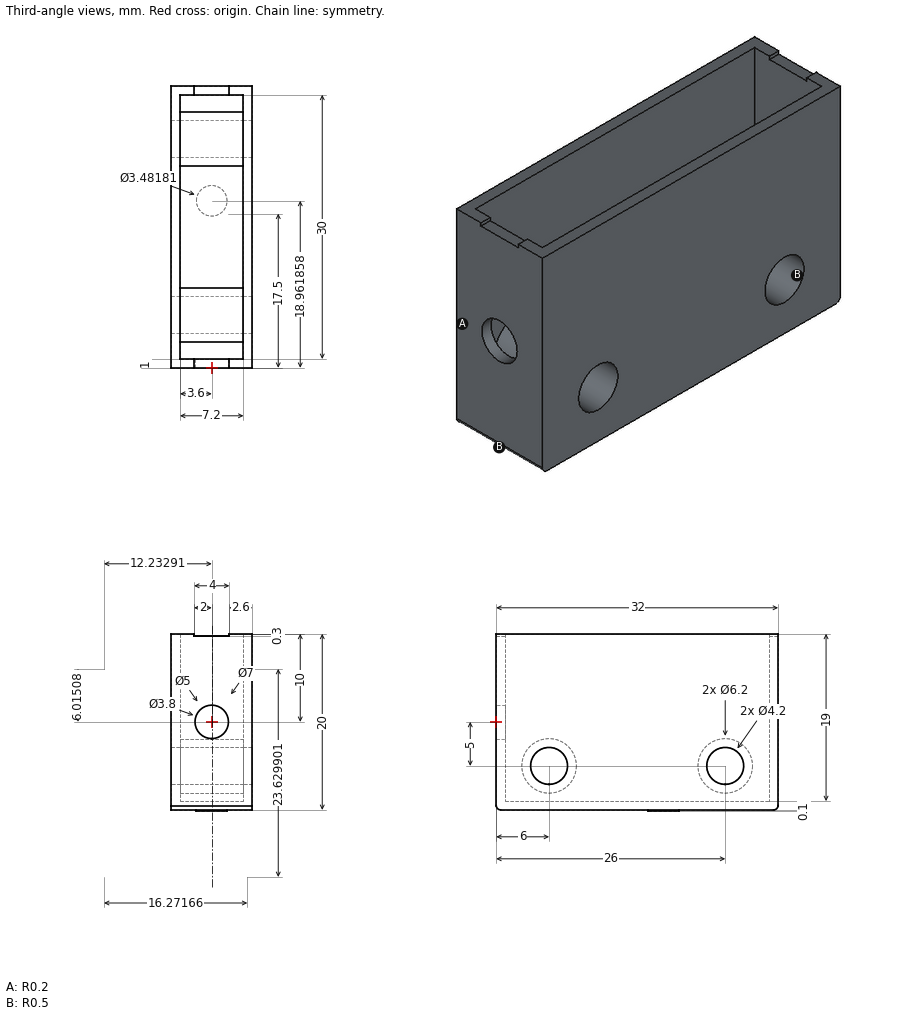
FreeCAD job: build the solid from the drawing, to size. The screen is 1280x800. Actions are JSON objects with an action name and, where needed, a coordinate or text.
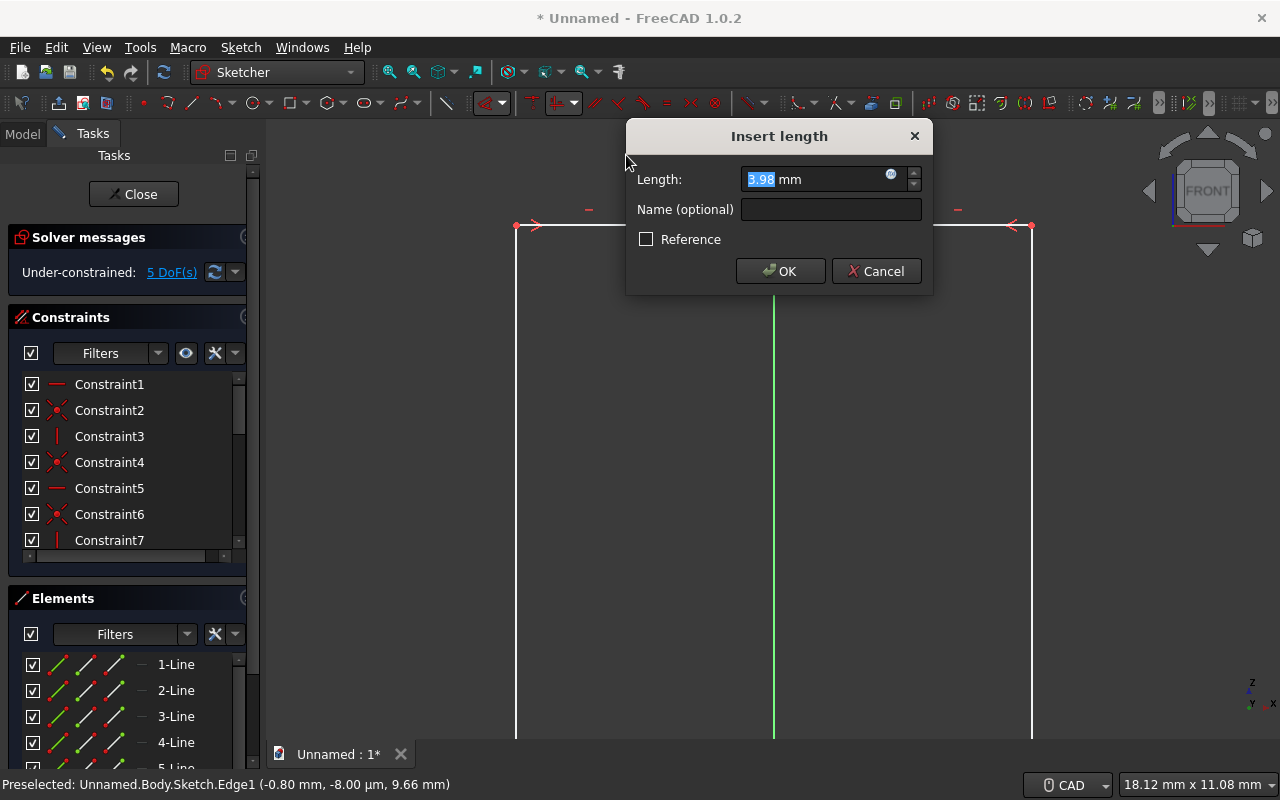
{"action": "type", "text": "4"}
{"action": "key", "text": "Return"}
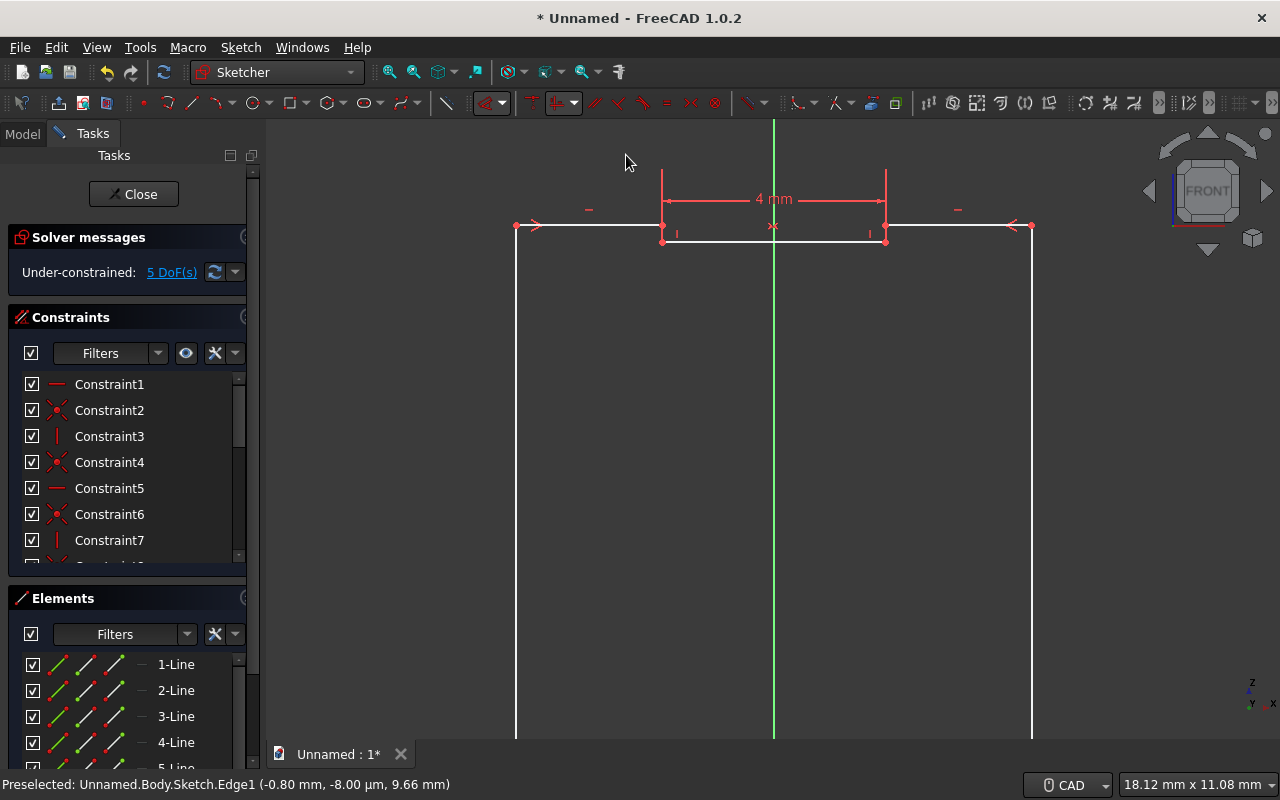
{"action": "left_click", "coordinate": [1032, 561]}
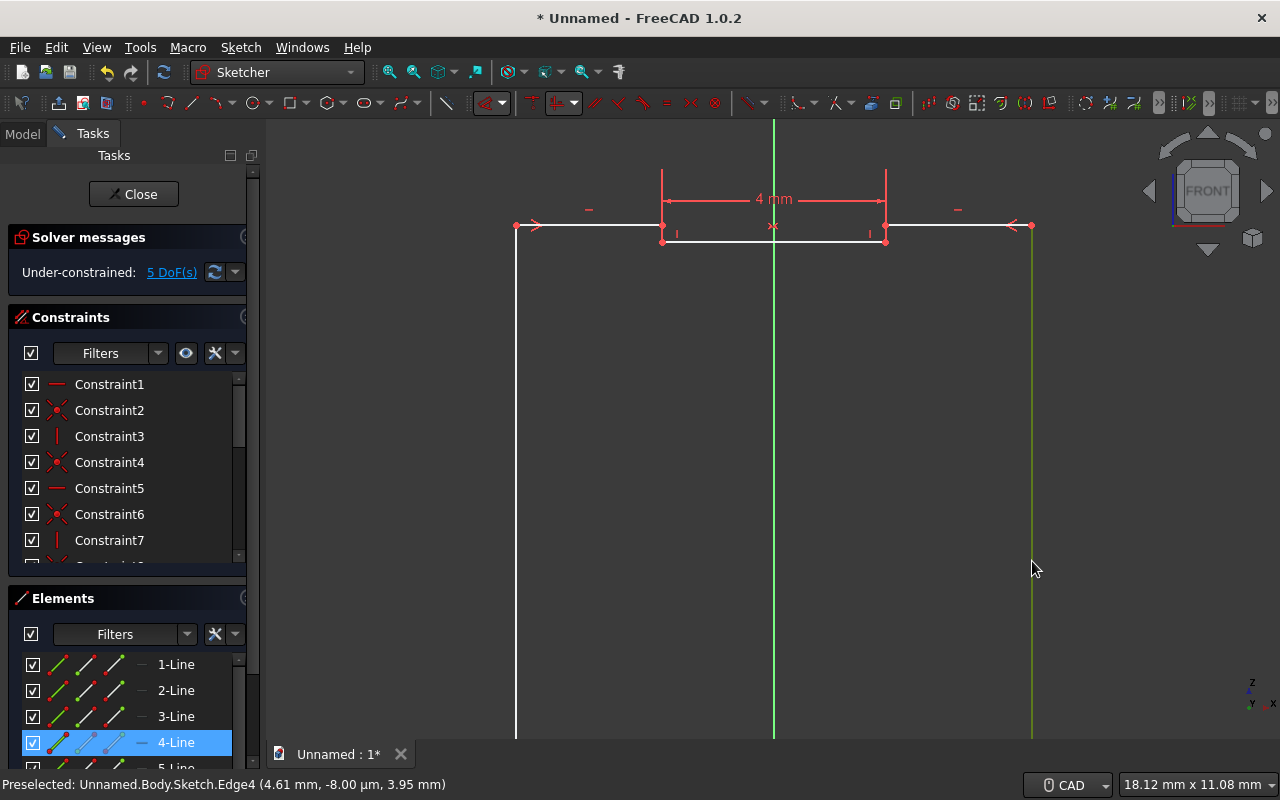
{"action": "key", "text": "i"}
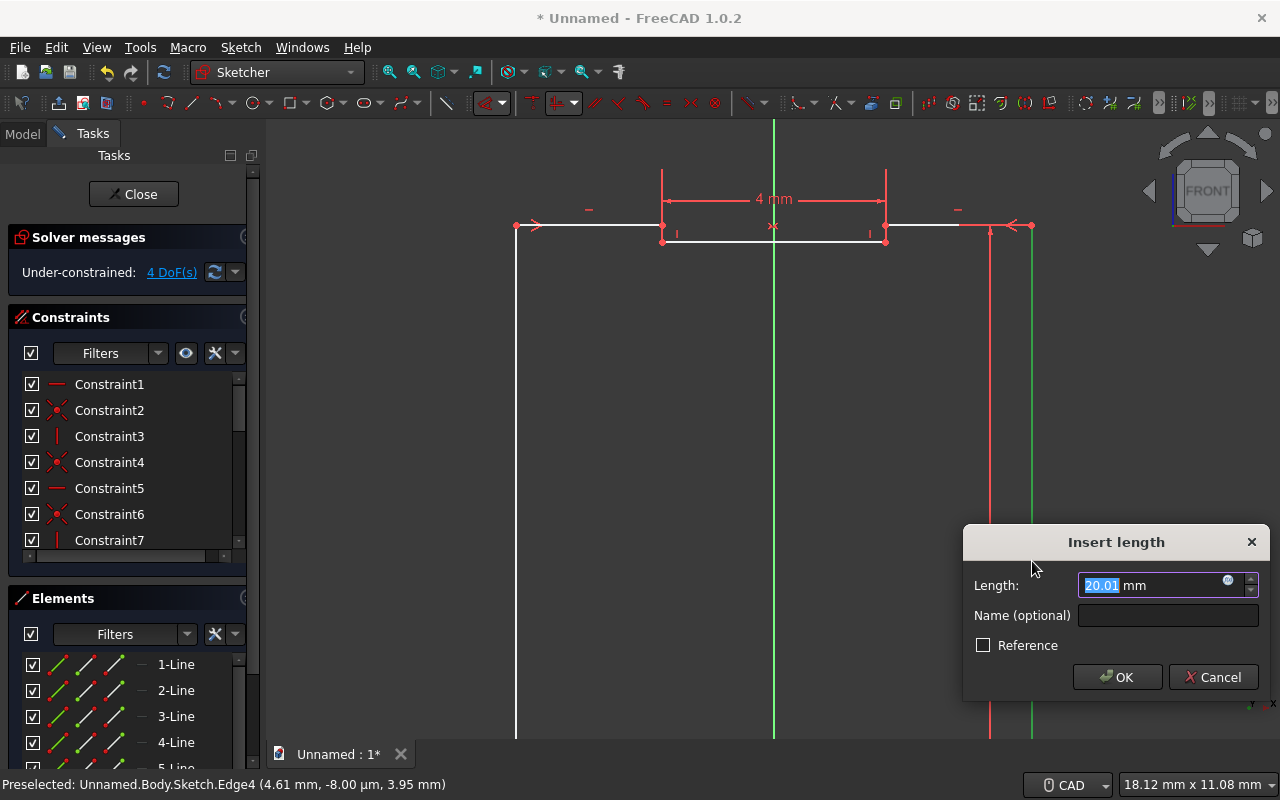
{"action": "type", "text": "20"}
{"action": "key", "text": "Return"}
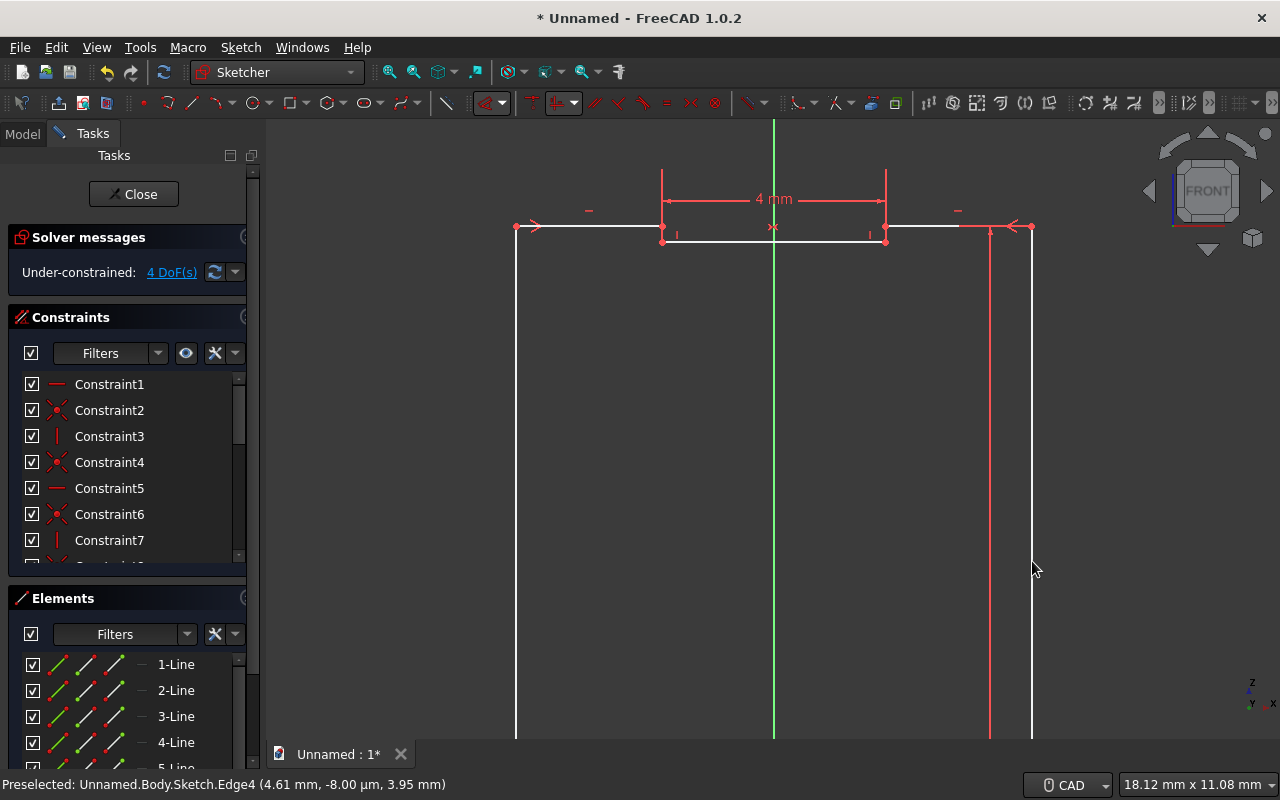
{"action": "left_click", "coordinate": [662, 242]}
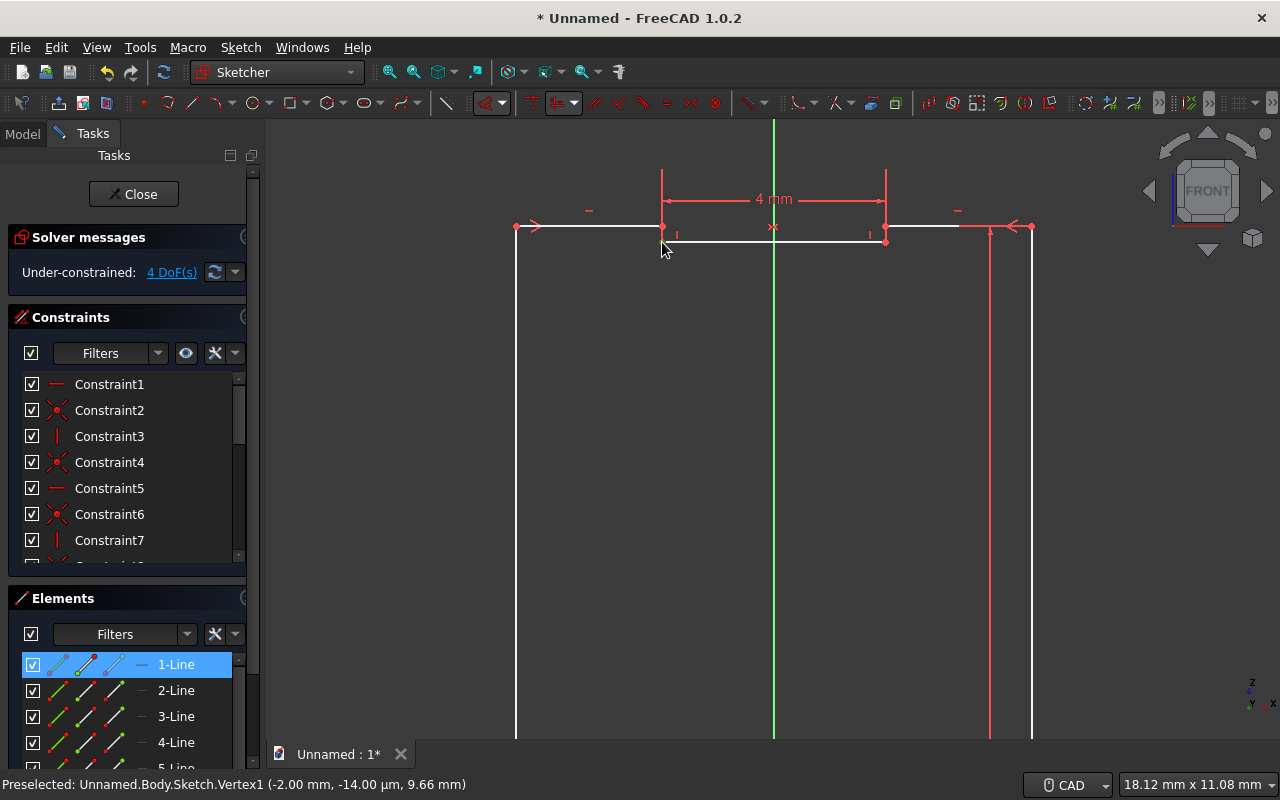
{"action": "left_click", "coordinate": [504, 104]}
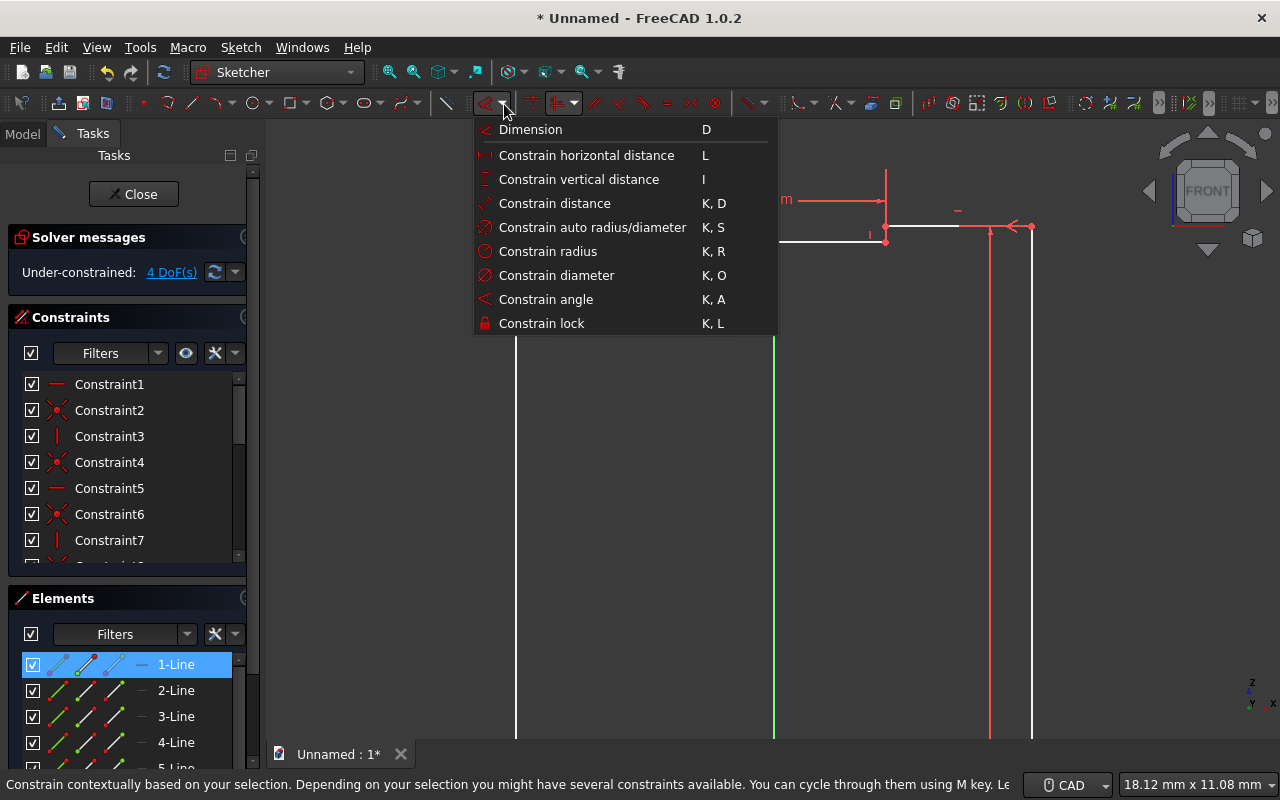
{"action": "left_click", "coordinate": [626, 155]}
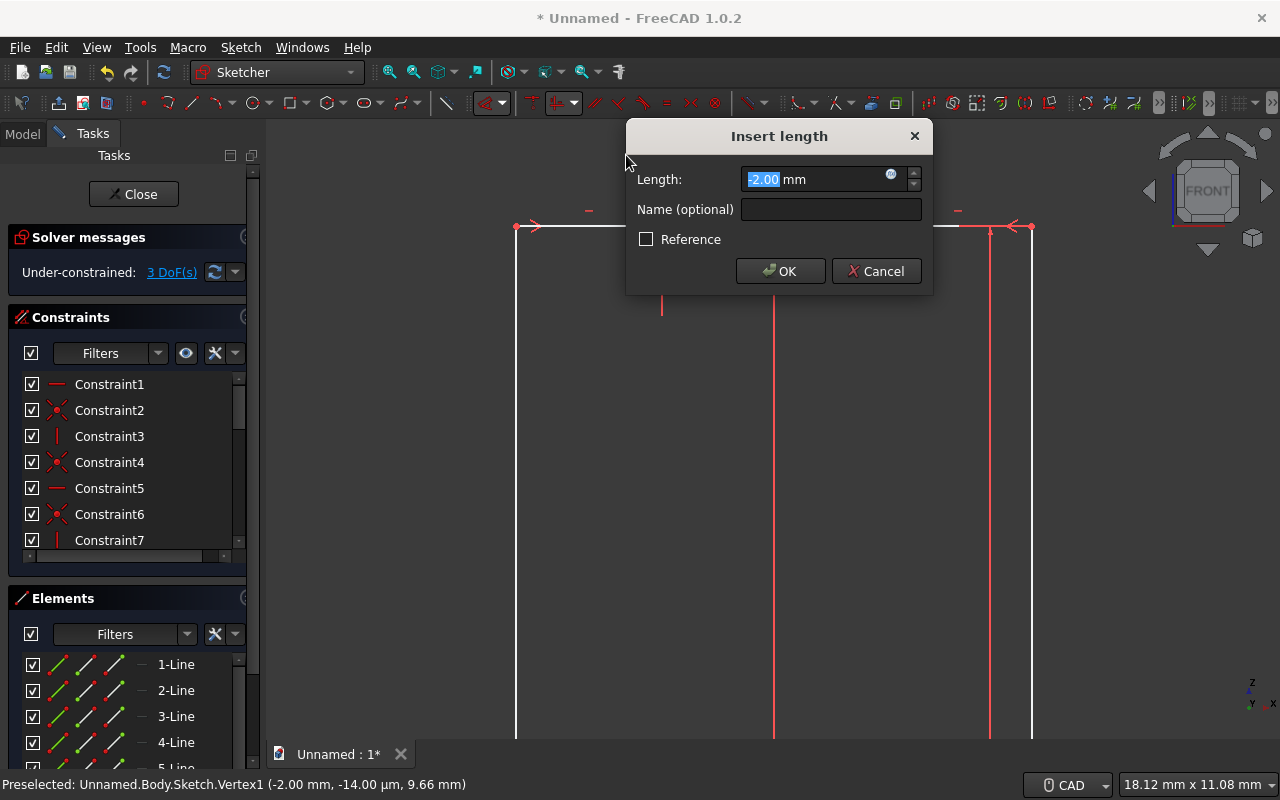
{"action": "type", "text": "-2"}
{"action": "key", "text": "Return"}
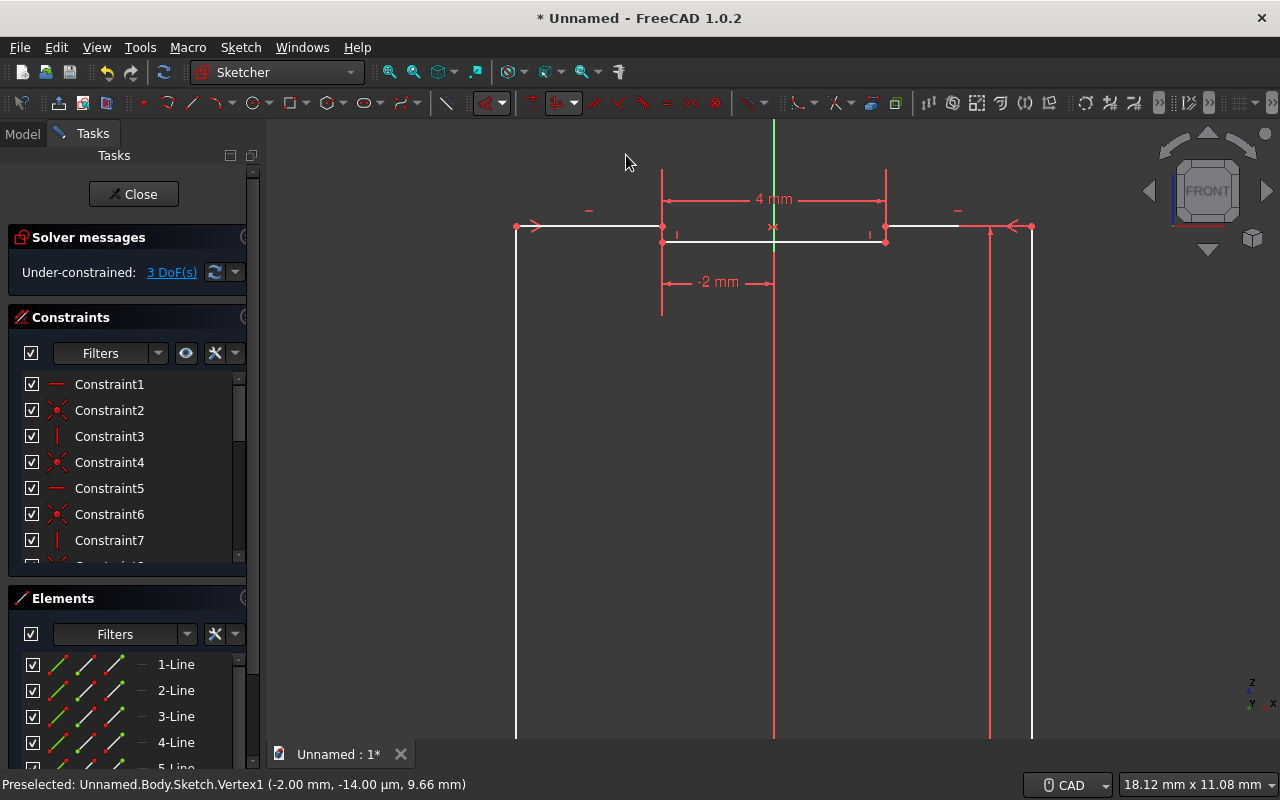
{"action": "scroll", "coordinate": [886, 234], "scroll_direction": "up", "scroll_amount": 5}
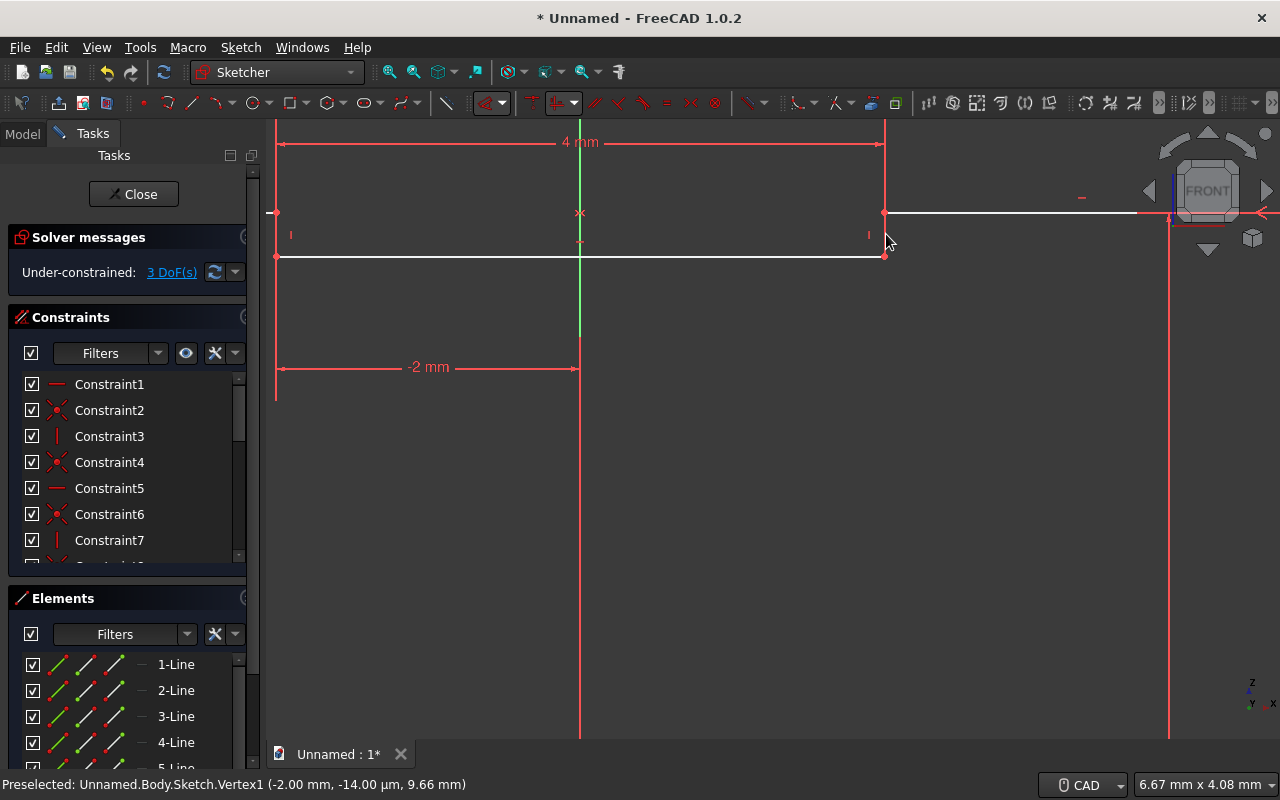
{"action": "left_click", "coordinate": [885, 235]}